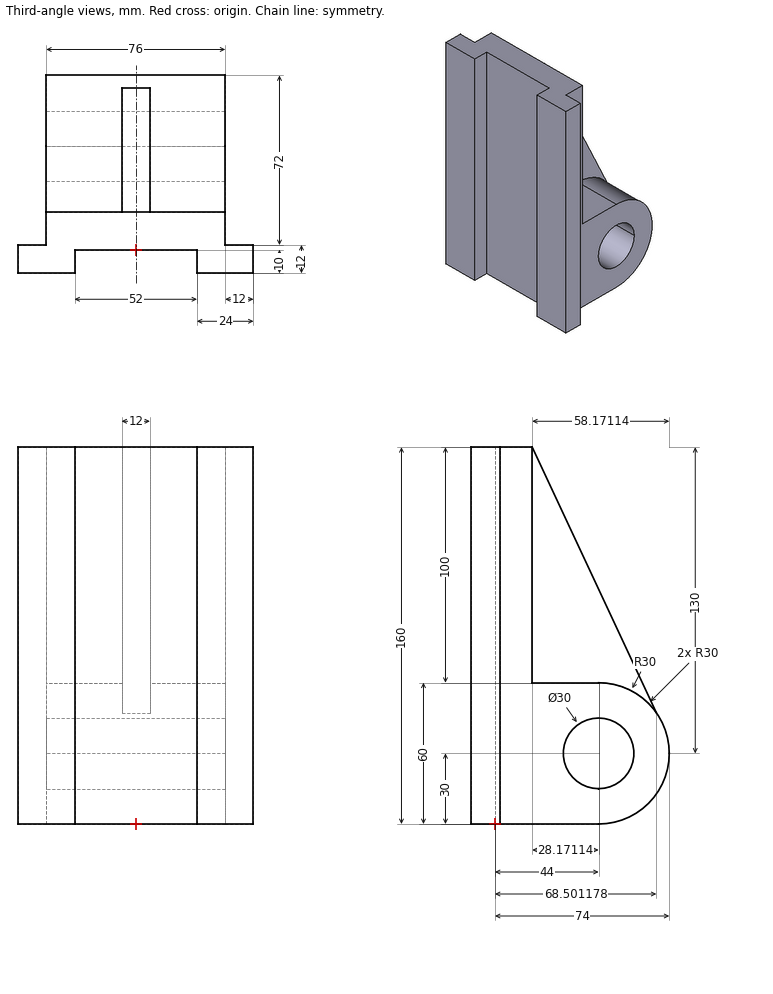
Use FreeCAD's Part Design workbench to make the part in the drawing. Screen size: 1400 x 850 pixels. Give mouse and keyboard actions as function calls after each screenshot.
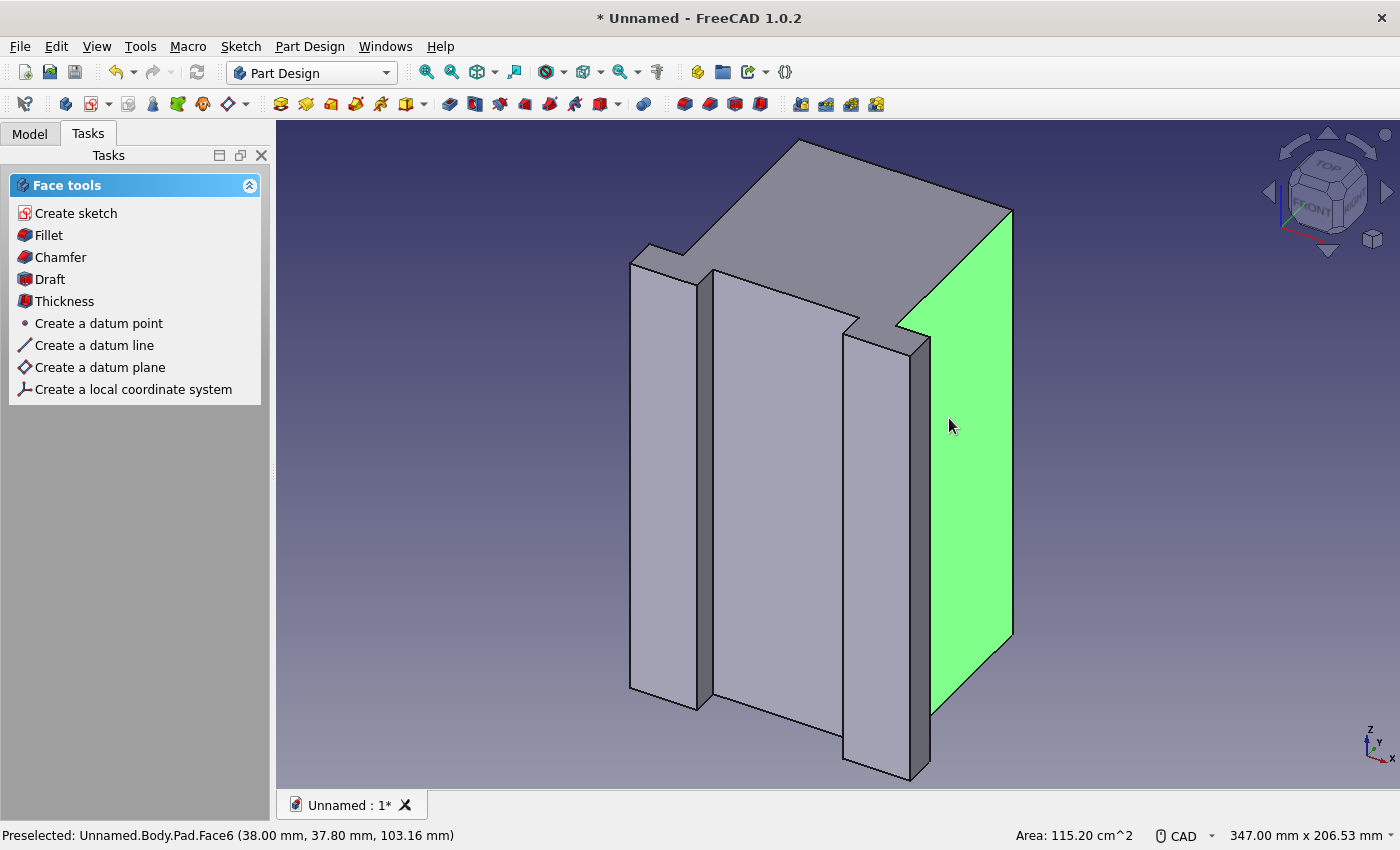
click(90, 104)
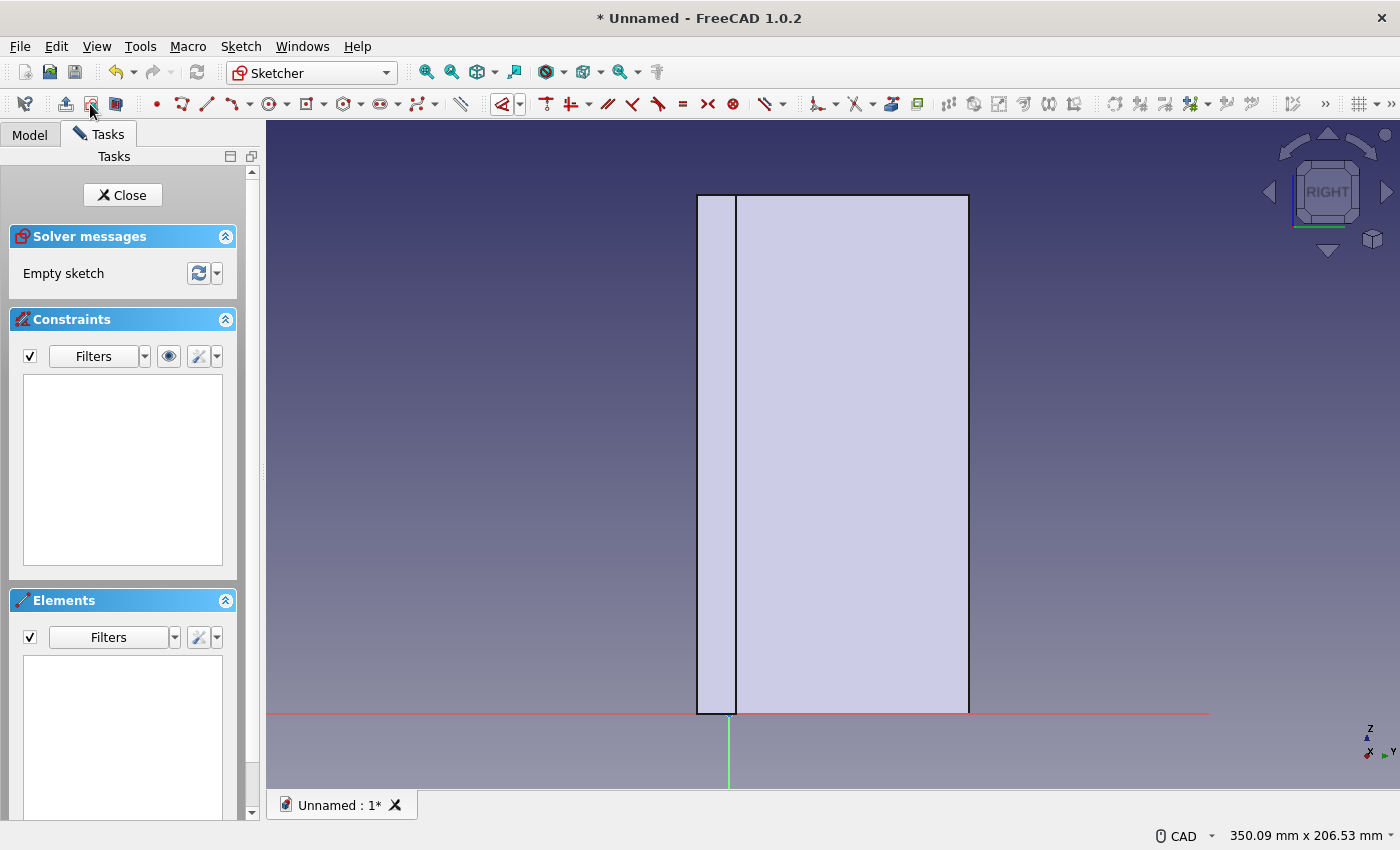
key(g)
key(m)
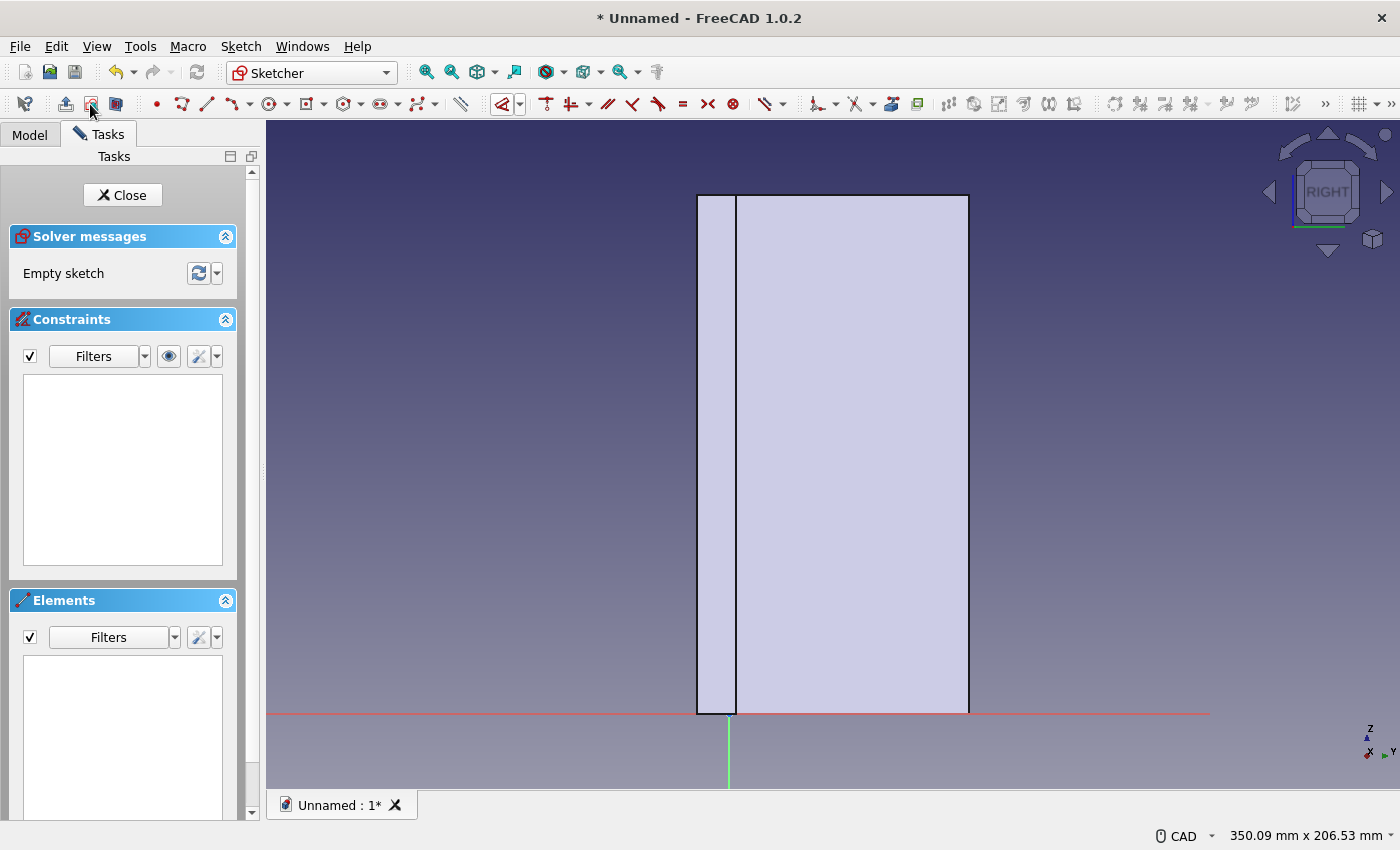
click(969, 616)
click(969, 195)
click(781, 195)
click(781, 519)
click(872, 519)
right_click(872, 519)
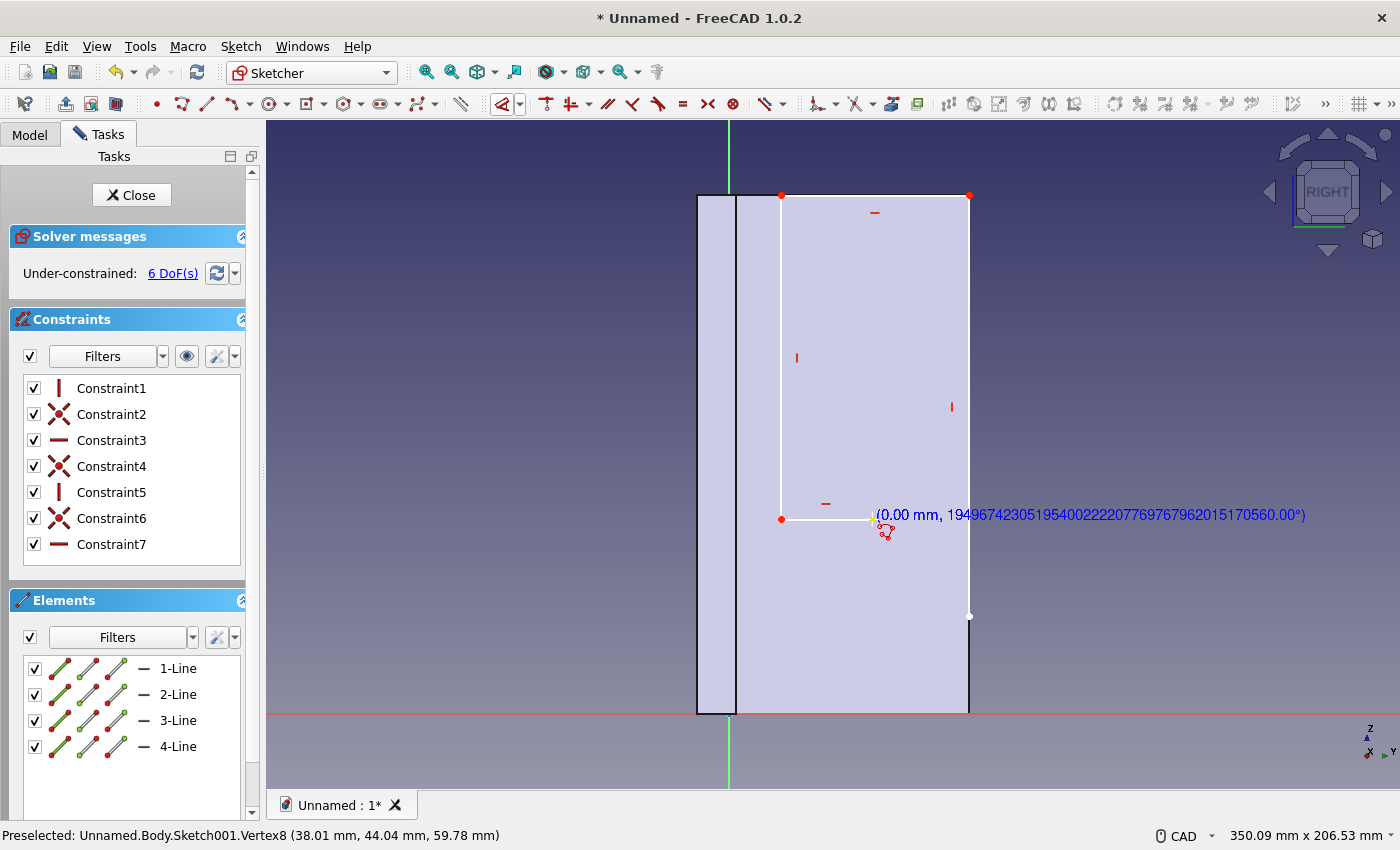
click(232, 104)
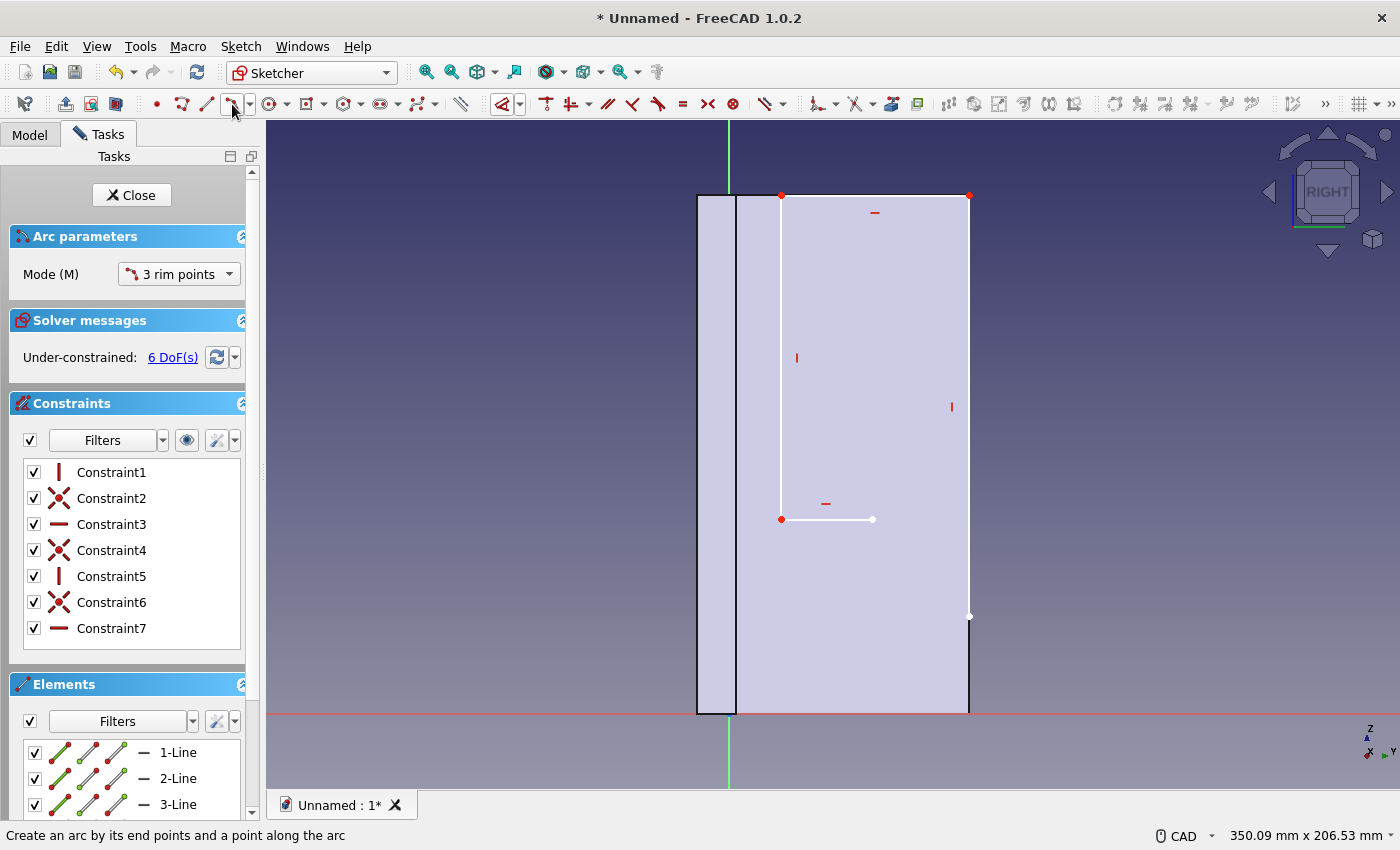
click(872, 520)
click(969, 617)
click(941, 548)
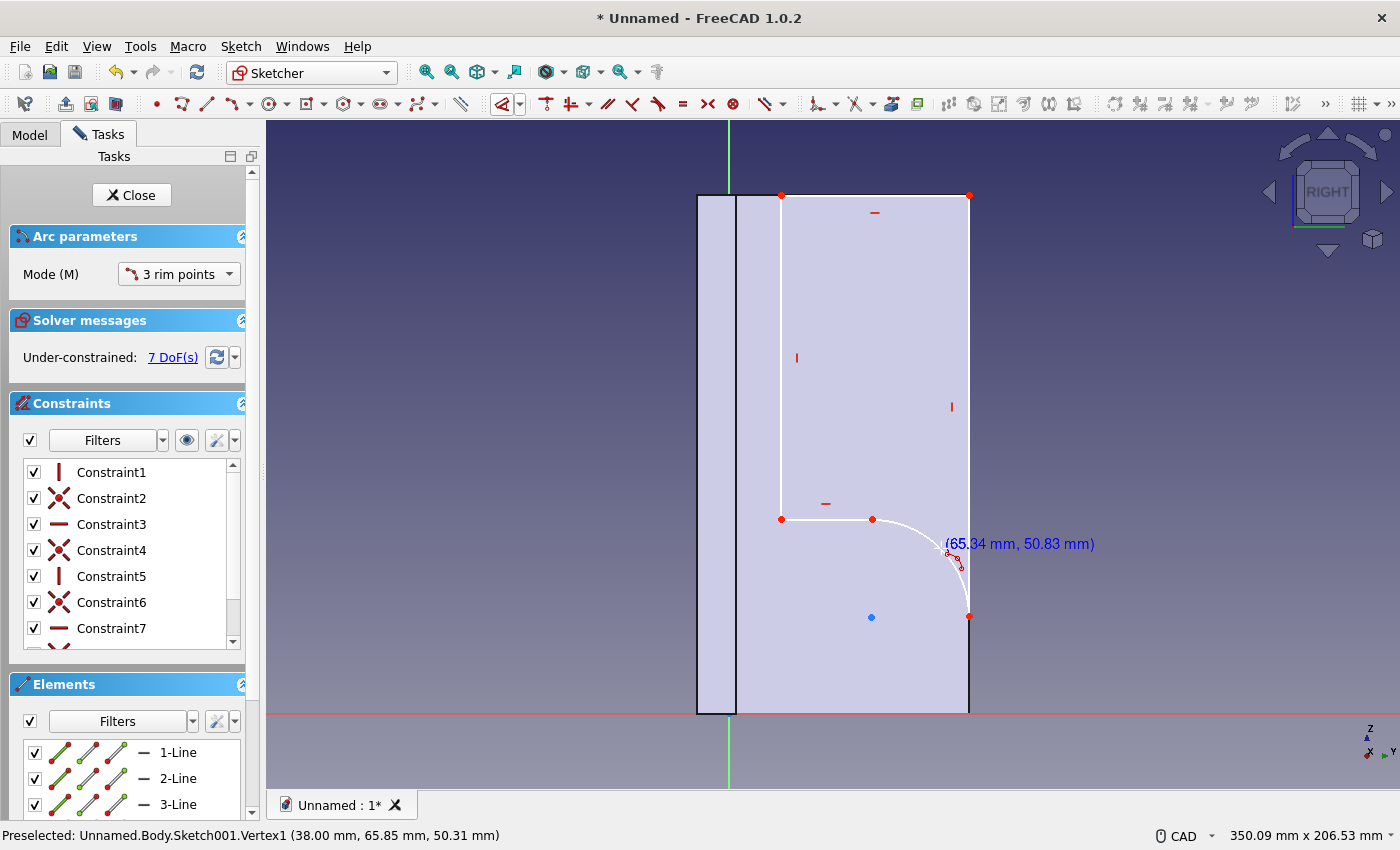
key(g)
key(m)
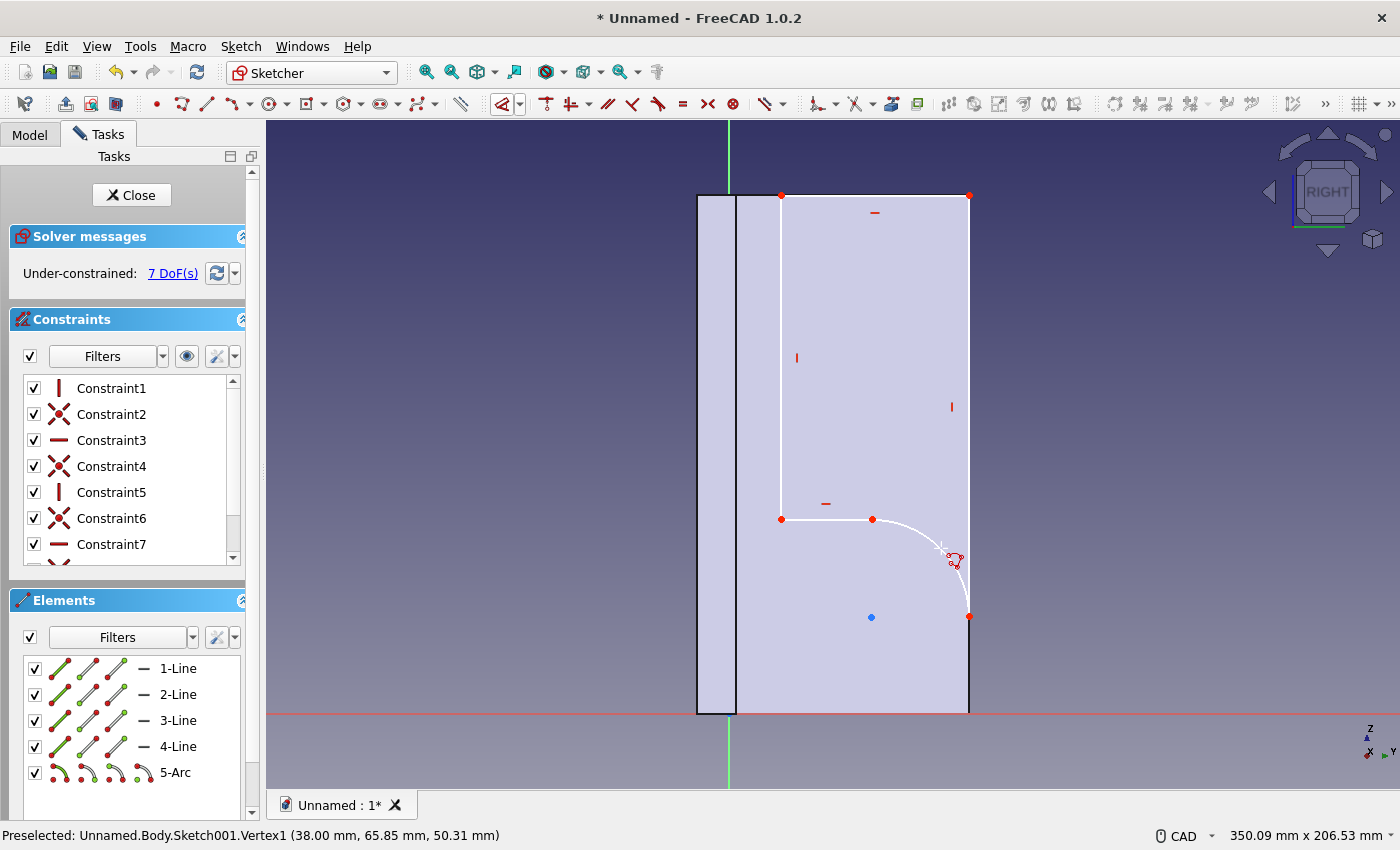
click(872, 714)
click(969, 705)
click(969, 617)
right_click(969, 705)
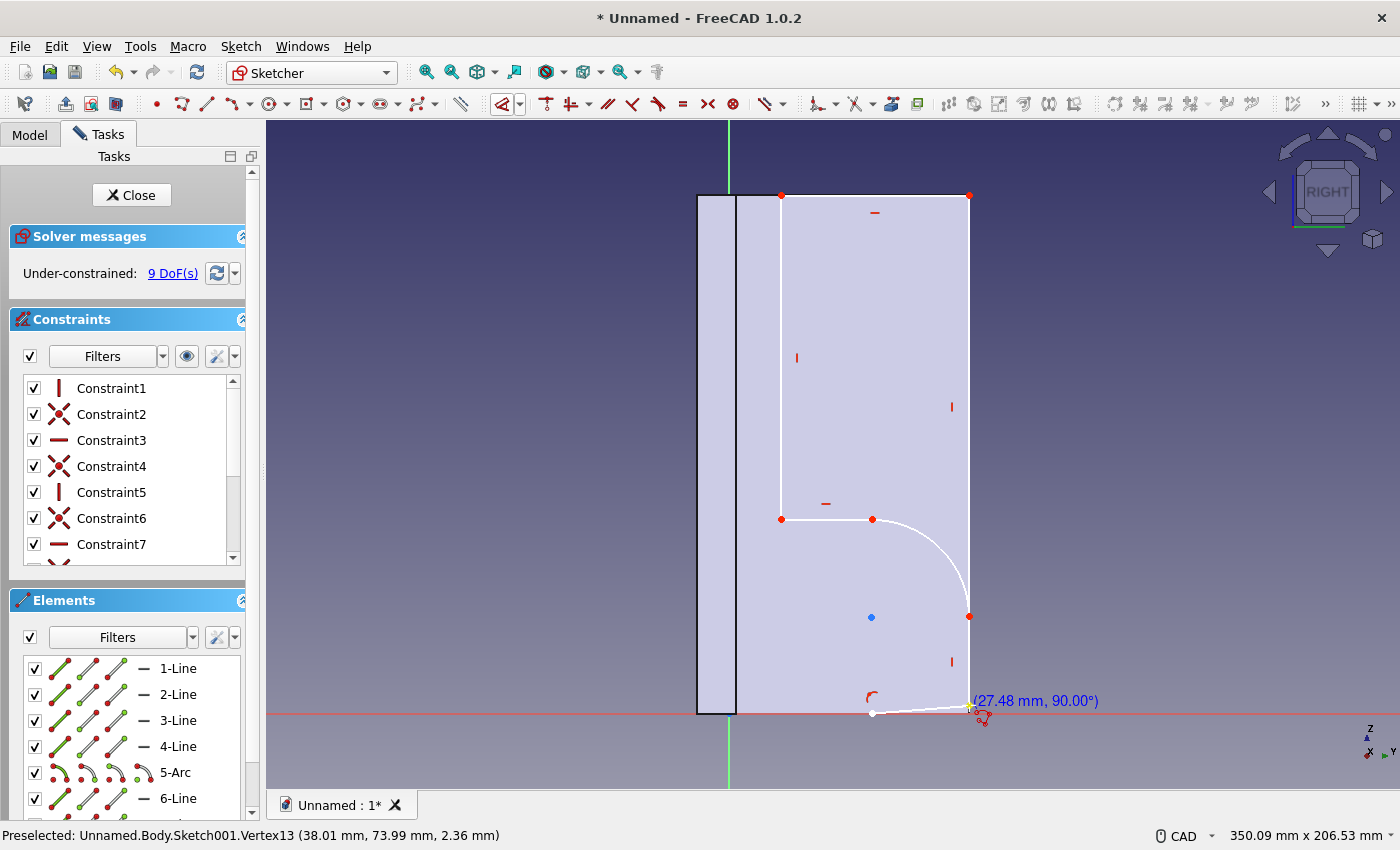
click(232, 104)